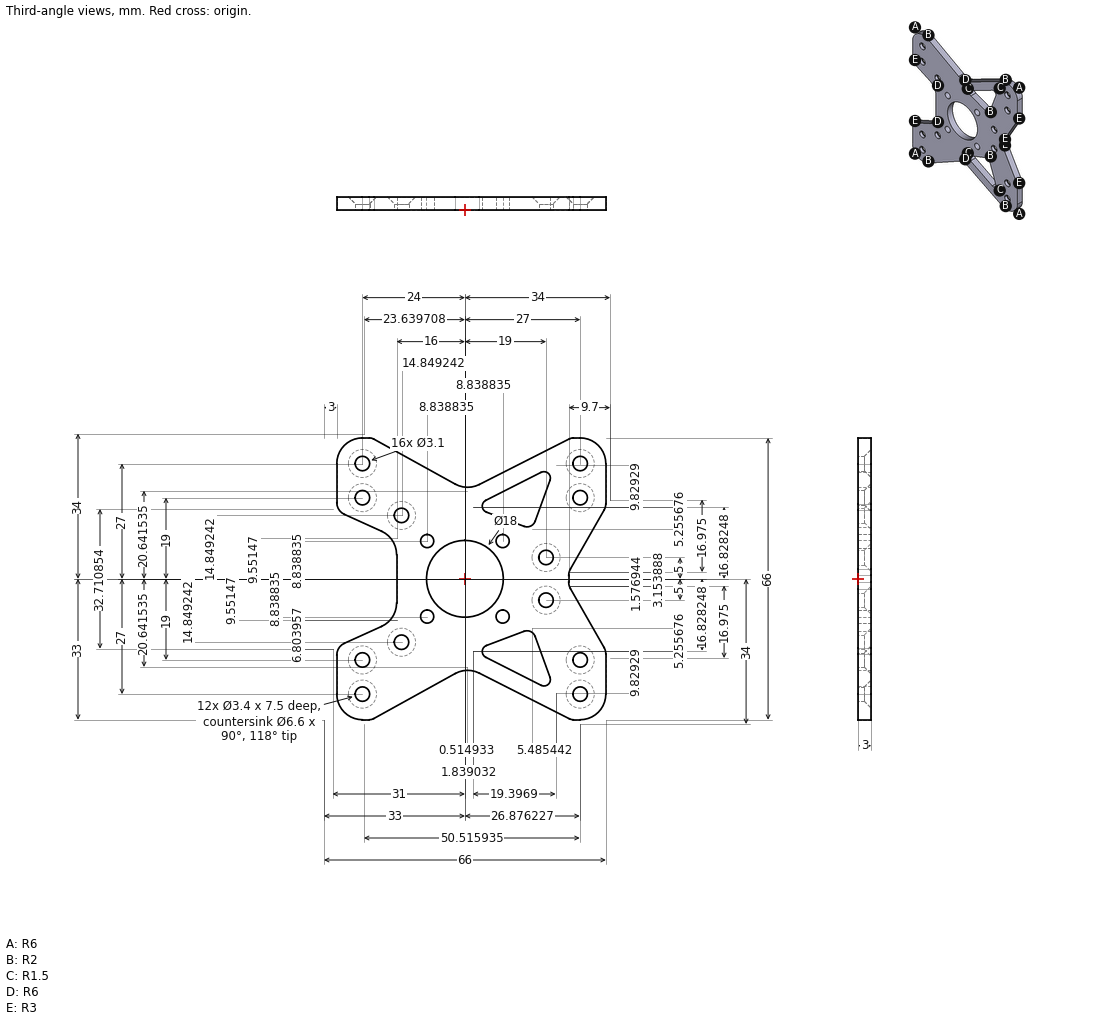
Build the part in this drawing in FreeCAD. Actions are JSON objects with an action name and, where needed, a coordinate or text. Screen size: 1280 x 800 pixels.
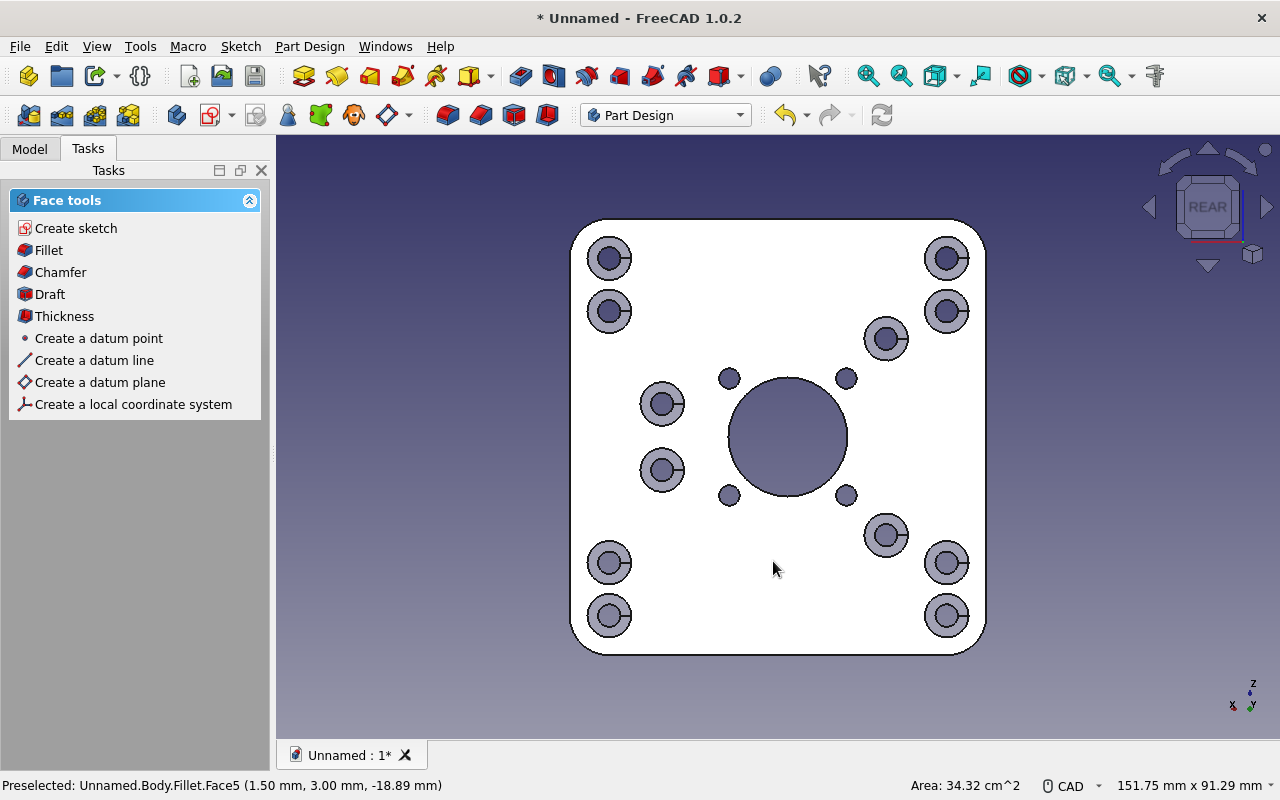
{"action": "left_click", "coordinate": [210, 116]}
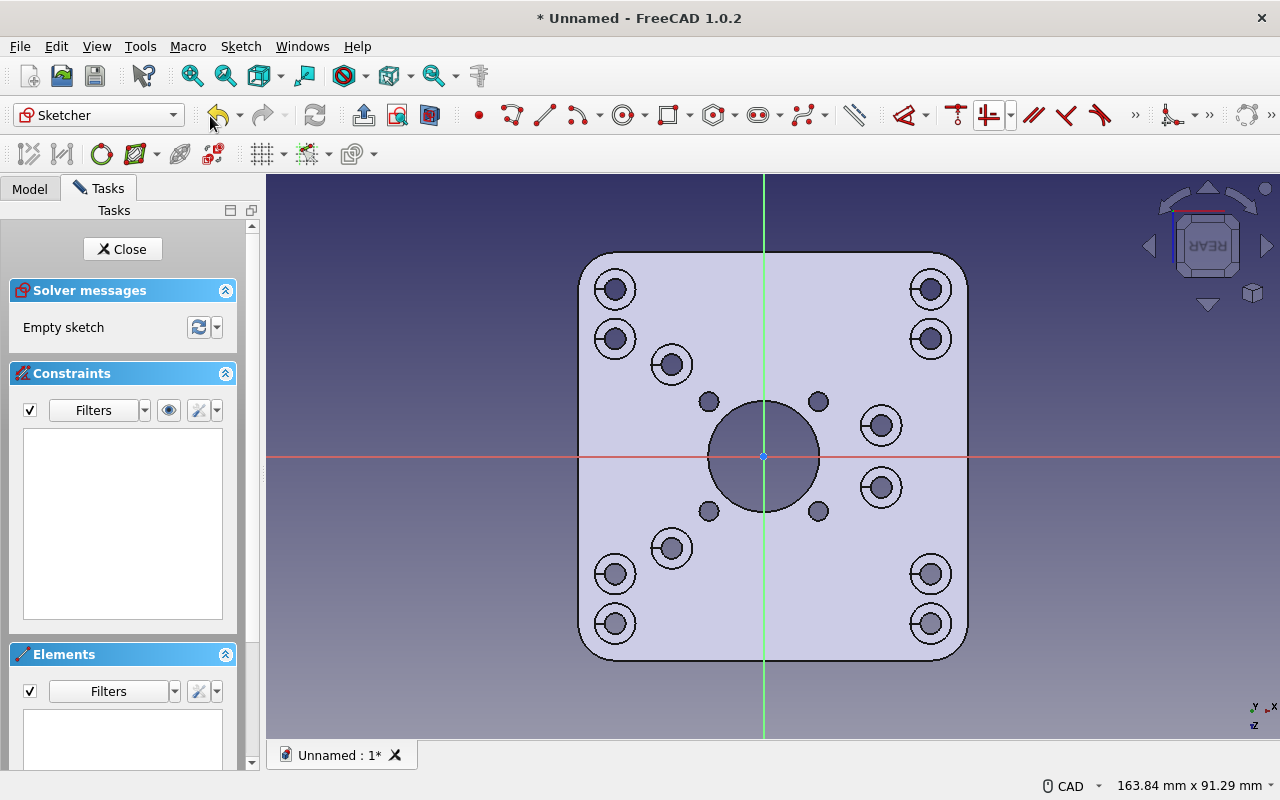
{"action": "key", "text": "g m"}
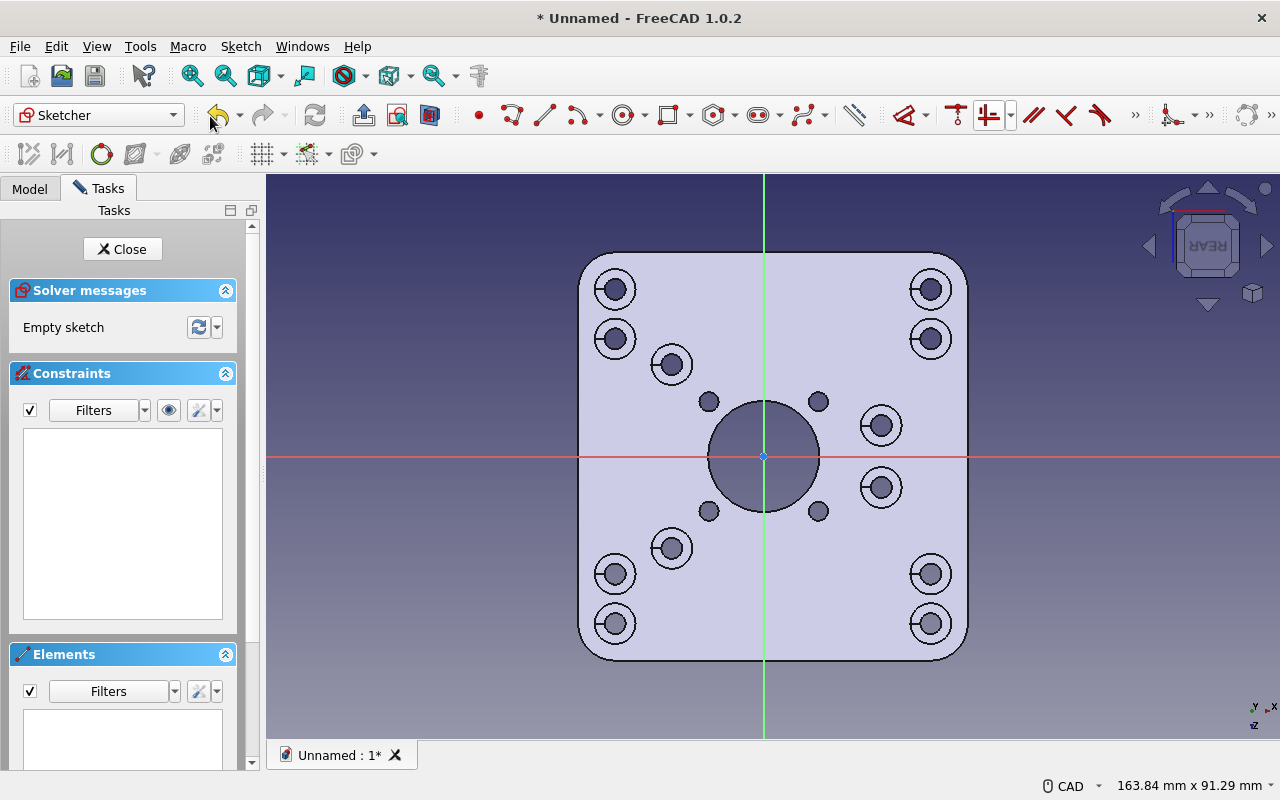
{"action": "left_click", "coordinate": [665, 516]}
{"action": "left_click", "coordinate": [665, 397]}
{"action": "left_click", "coordinate": [572, 355]}
{"action": "left_click", "coordinate": [572, 558]}
{"action": "left_click", "coordinate": [665, 517]}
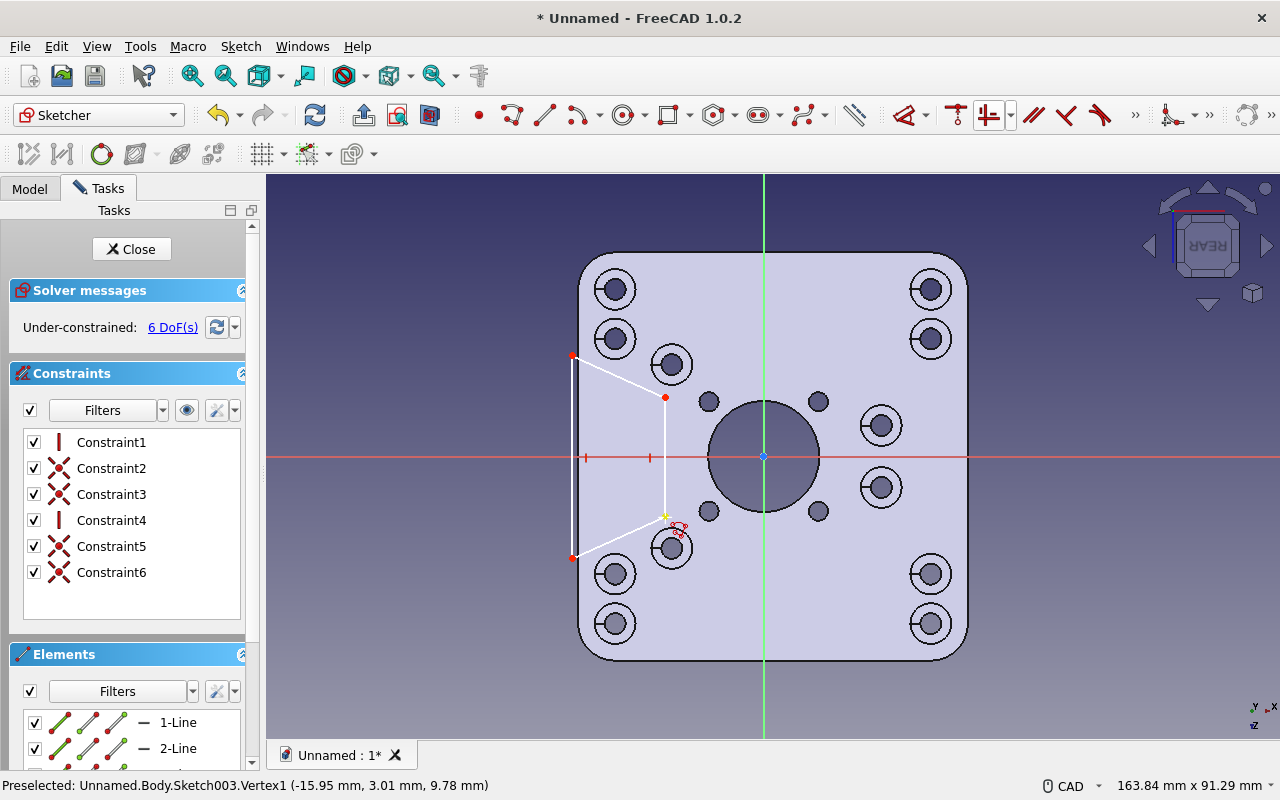
{"action": "scroll", "coordinate": [914, 447], "scroll_direction": "up", "scroll_amount": 3}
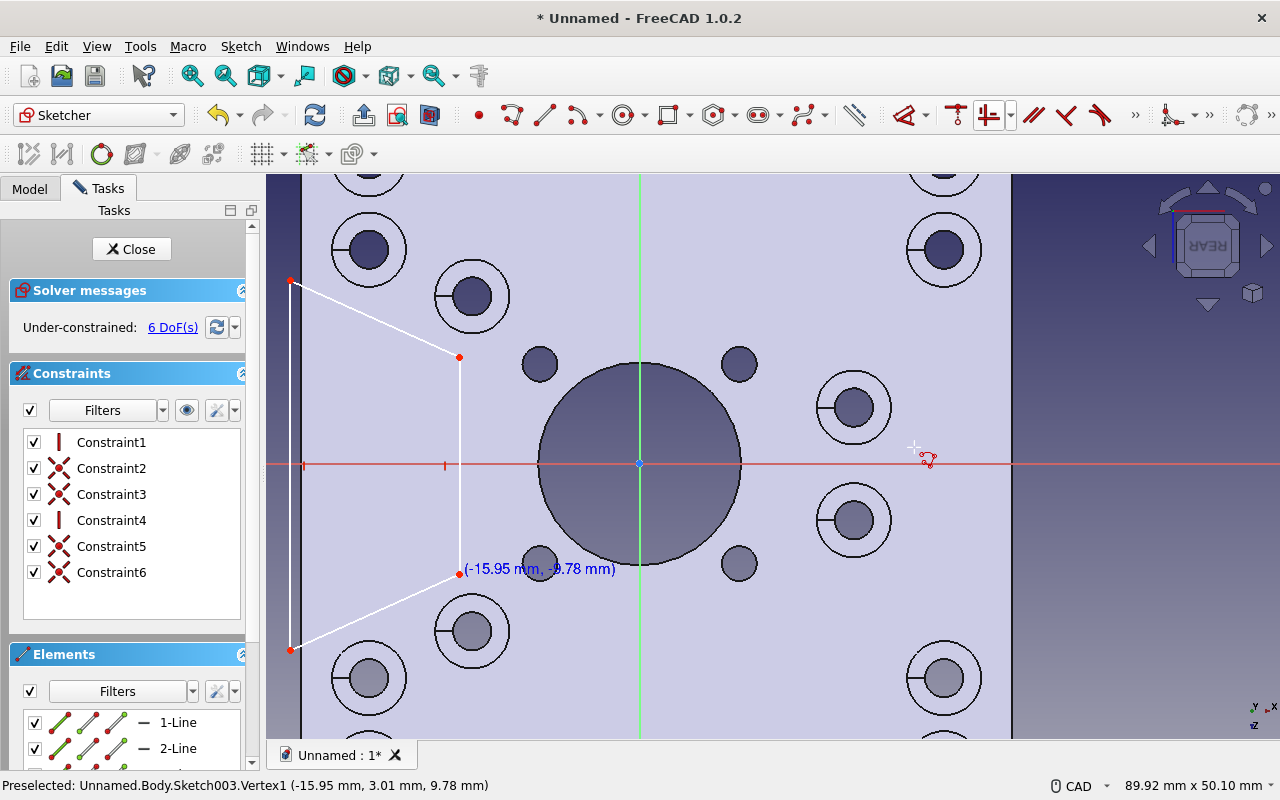
{"action": "left_click", "coordinate": [914, 446]}
{"action": "left_click", "coordinate": [914, 482]}
{"action": "left_click", "coordinate": [1023, 673]}
{"action": "left_click", "coordinate": [1023, 255]}
{"action": "left_click", "coordinate": [914, 447]}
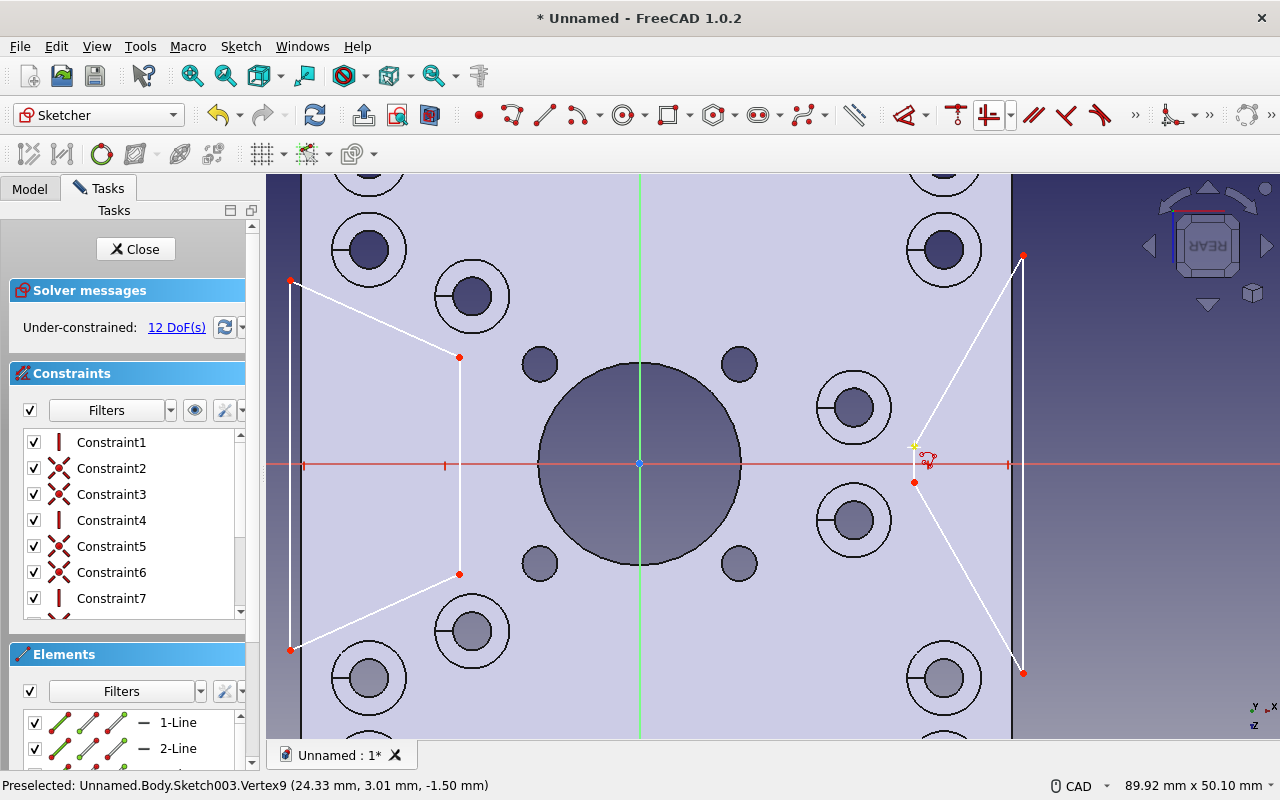
{"action": "scroll", "coordinate": [645, 231], "scroll_direction": "up", "scroll_amount": 6}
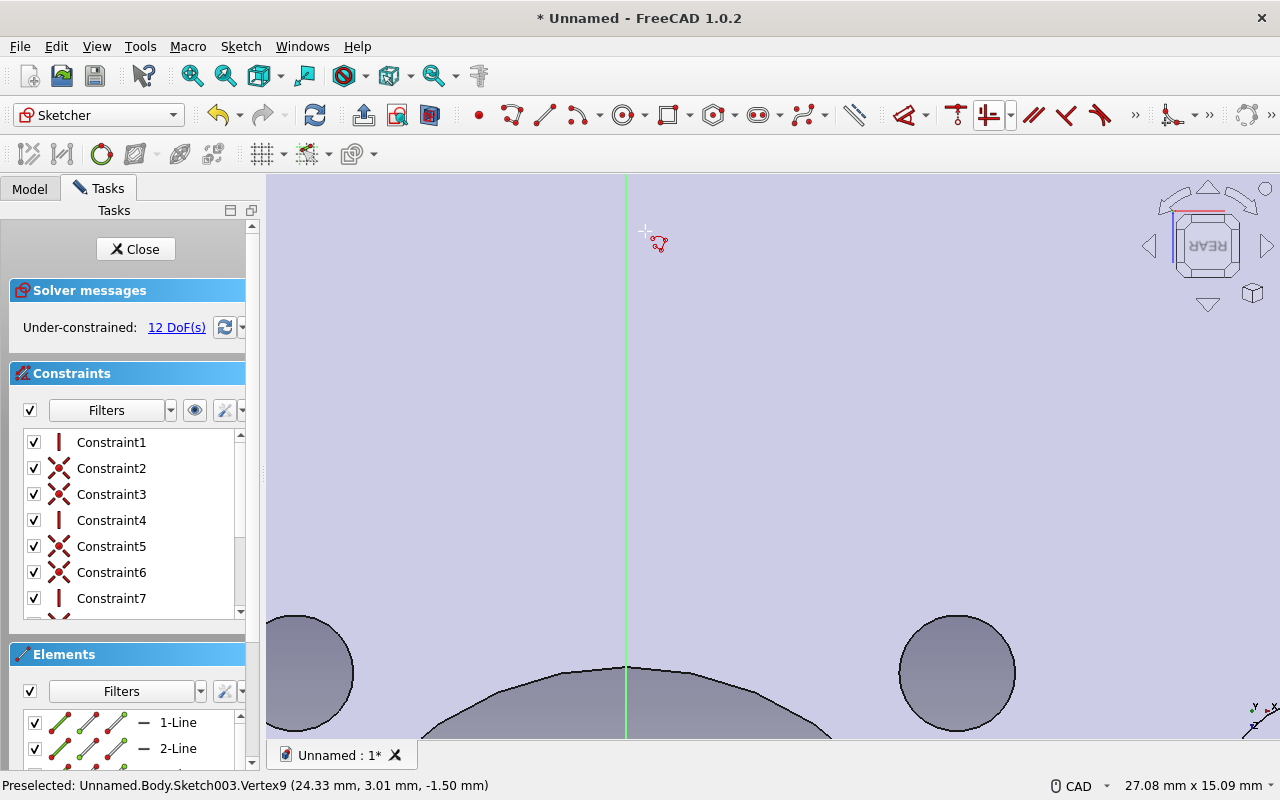
{"action": "left_click", "coordinate": [646, 231]}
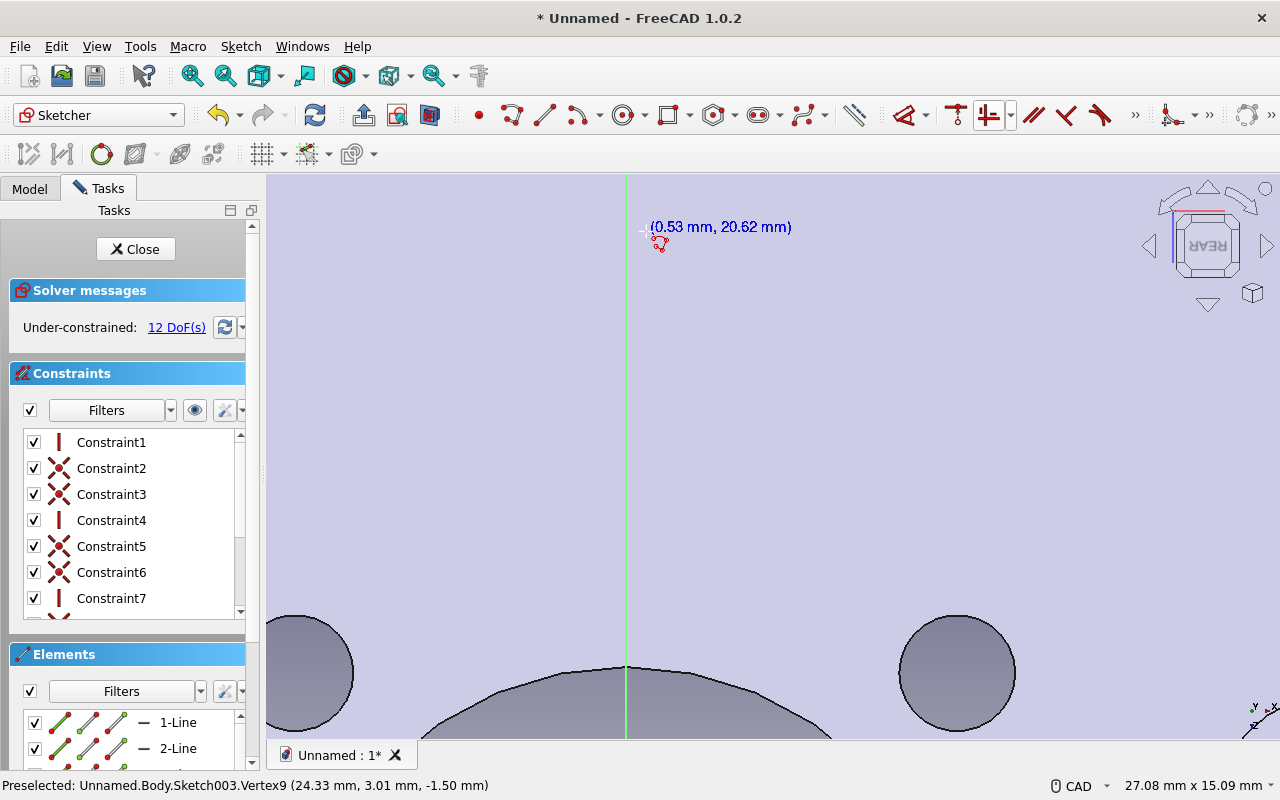
{"action": "scroll", "coordinate": [708, 371], "scroll_direction": "down", "scroll_amount": 10}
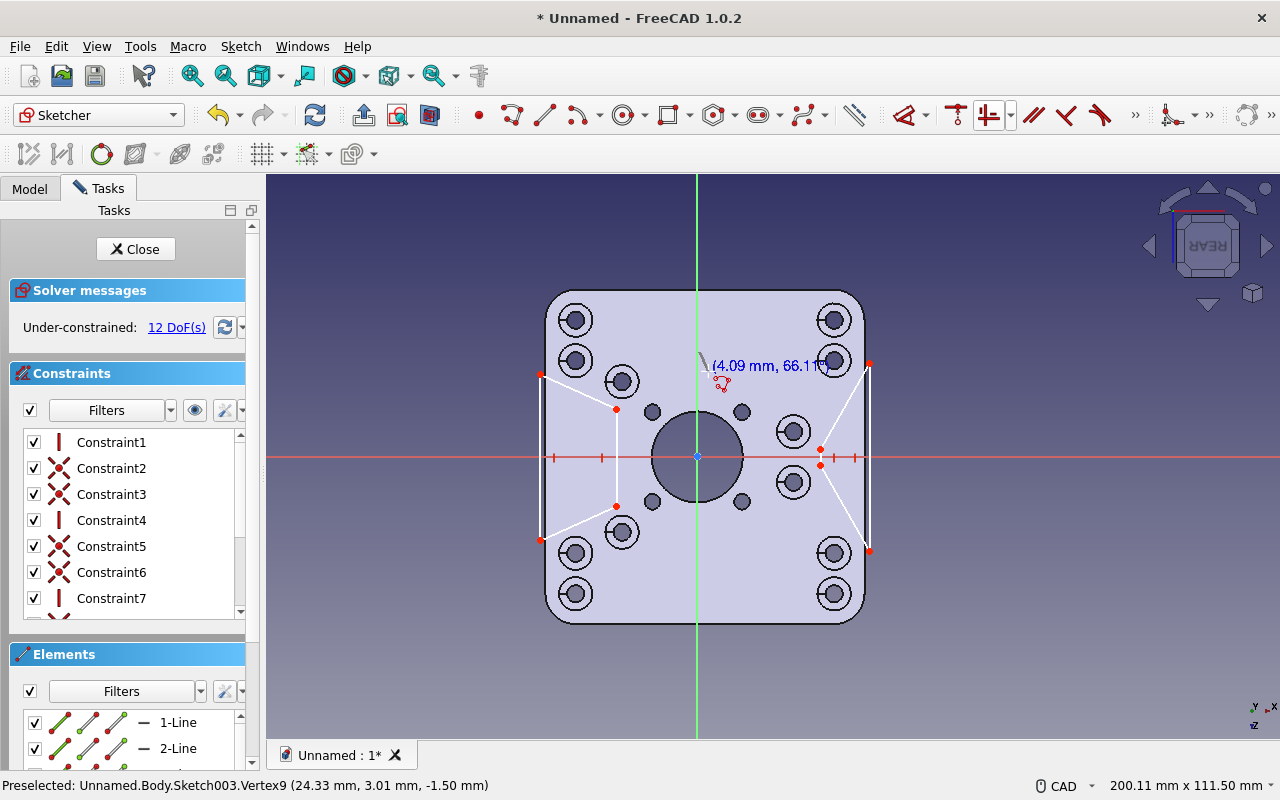
{"action": "left_click", "coordinate": [834, 285]}
{"action": "left_click", "coordinate": [578, 285]}